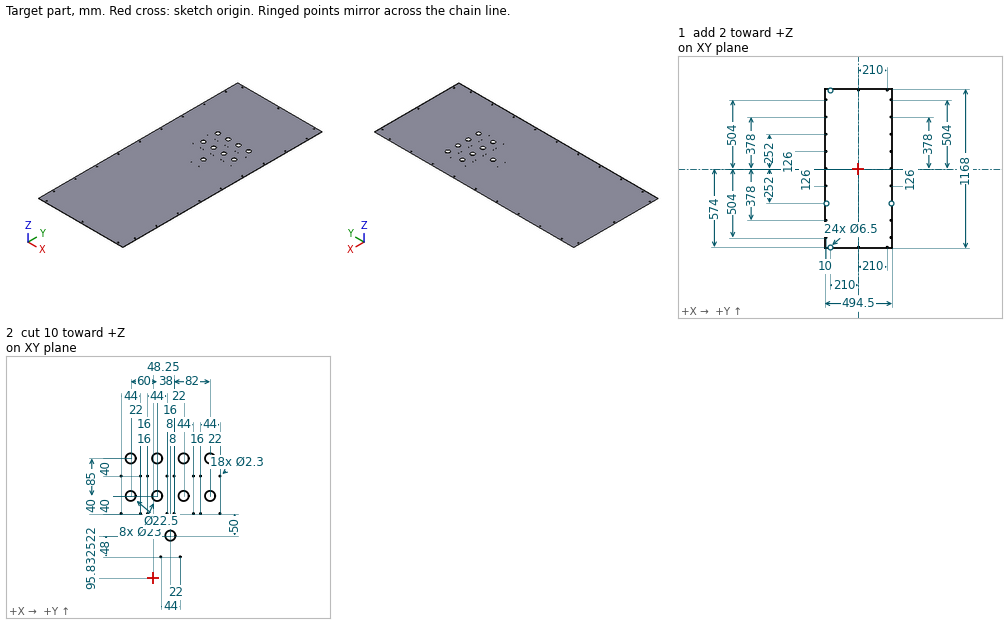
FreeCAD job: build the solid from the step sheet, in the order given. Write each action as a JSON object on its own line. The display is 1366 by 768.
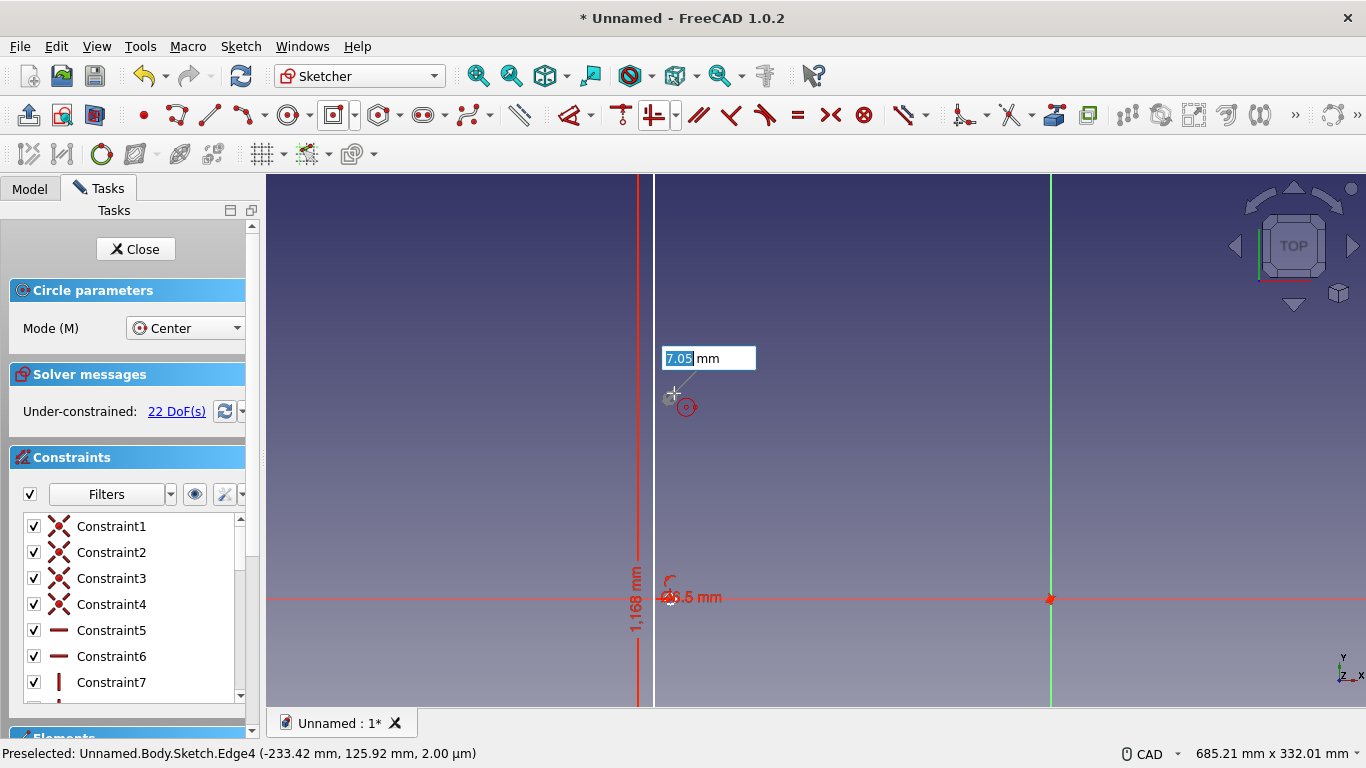
{"action": "type", "text": "6.5"}
{"action": "key", "text": "Return"}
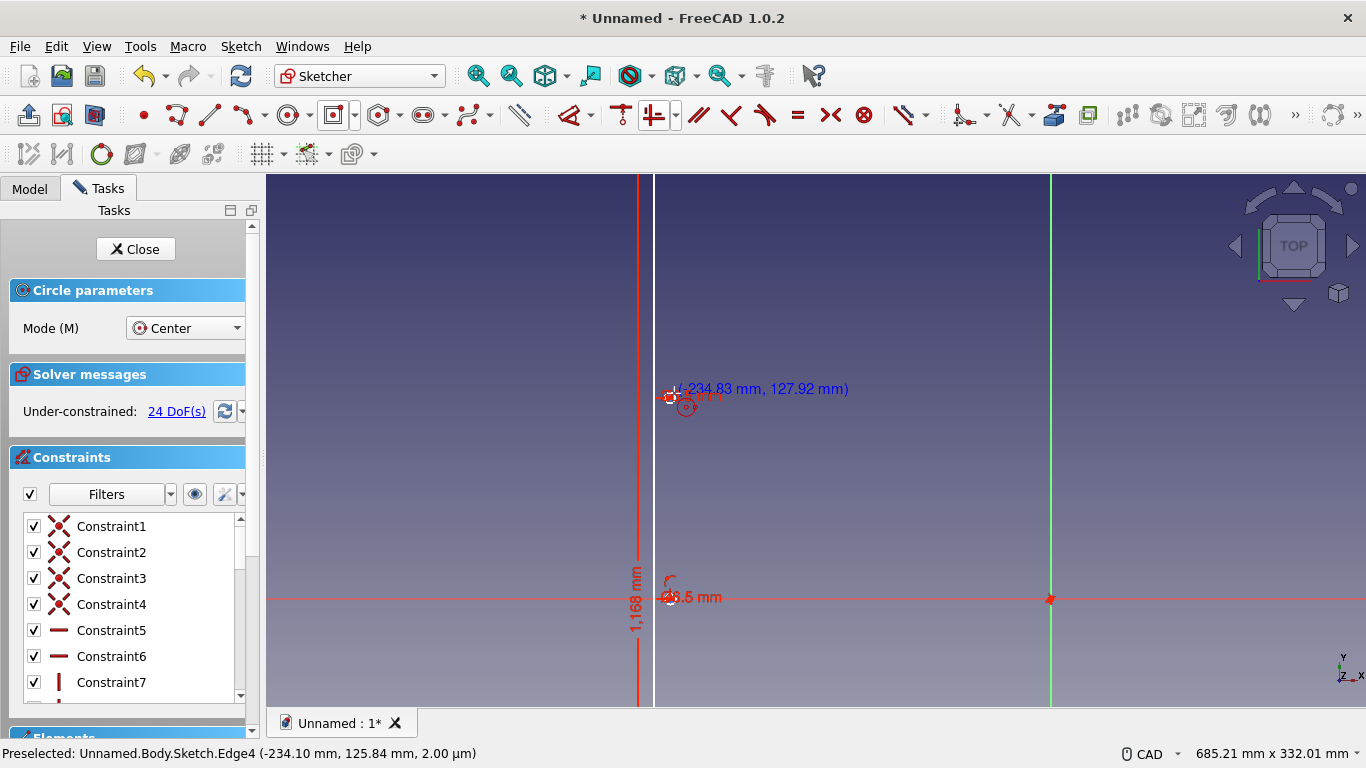
{"action": "scroll", "coordinate": [687, 409], "scroll_direction": "down", "scroll_amount": 9}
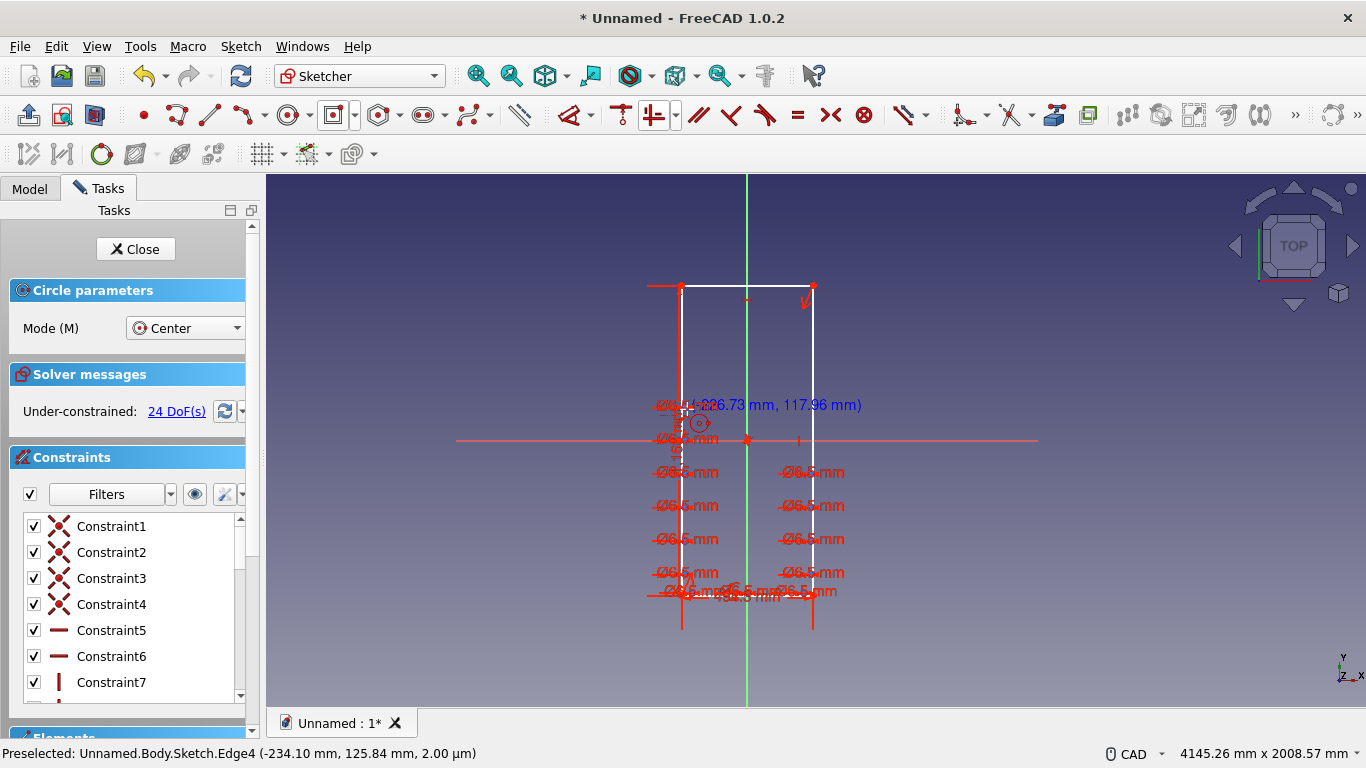
{"action": "scroll", "coordinate": [685, 374], "scroll_direction": "up", "scroll_amount": 17}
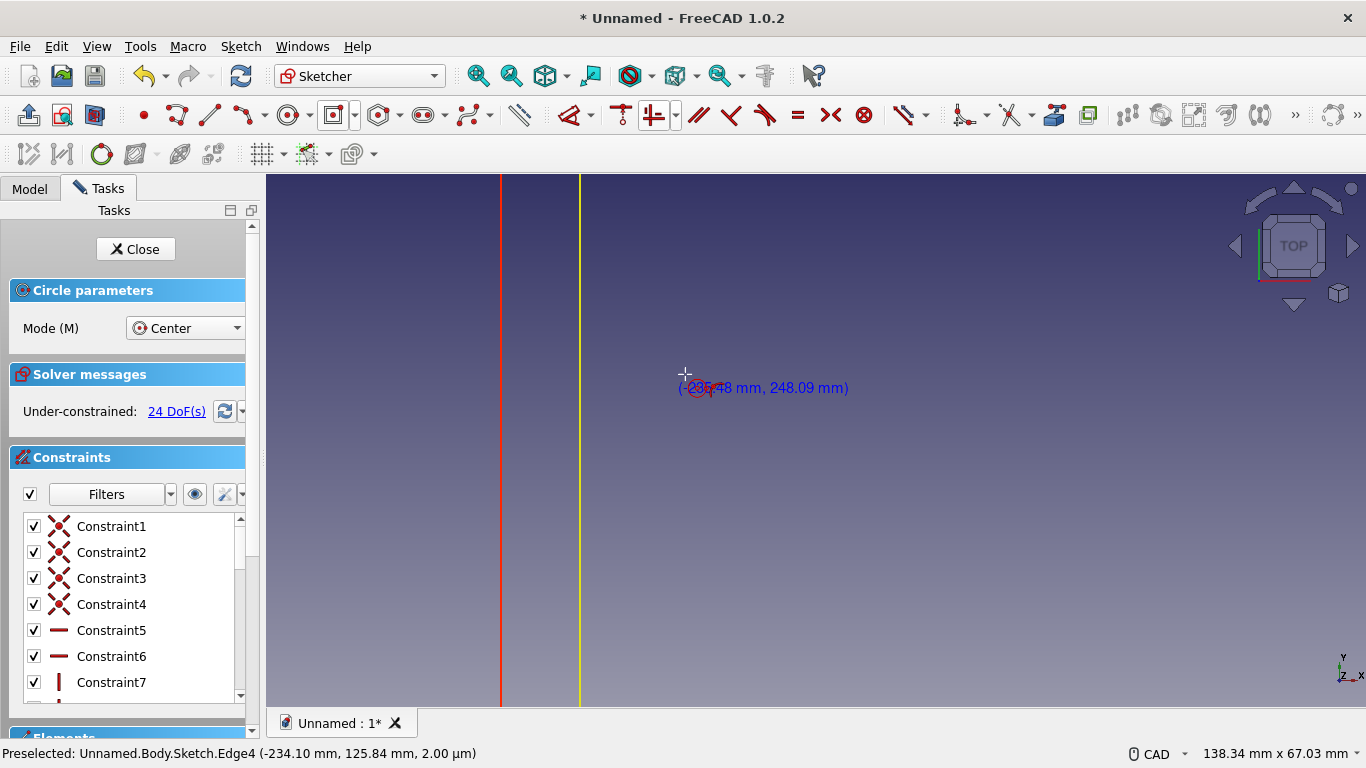
{"action": "scroll", "coordinate": [671, 359], "scroll_direction": "down", "scroll_amount": 16}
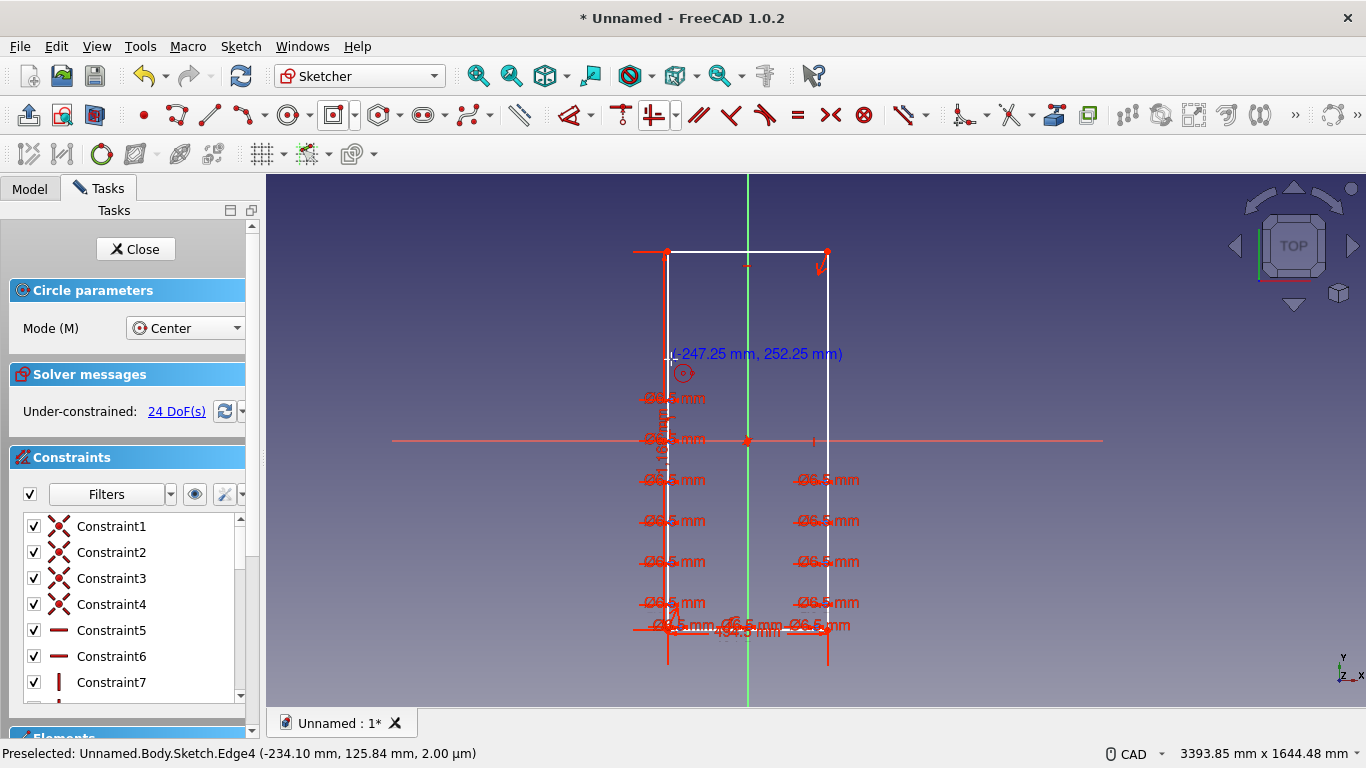
{"action": "scroll", "coordinate": [671, 359], "scroll_direction": "up", "scroll_amount": 8}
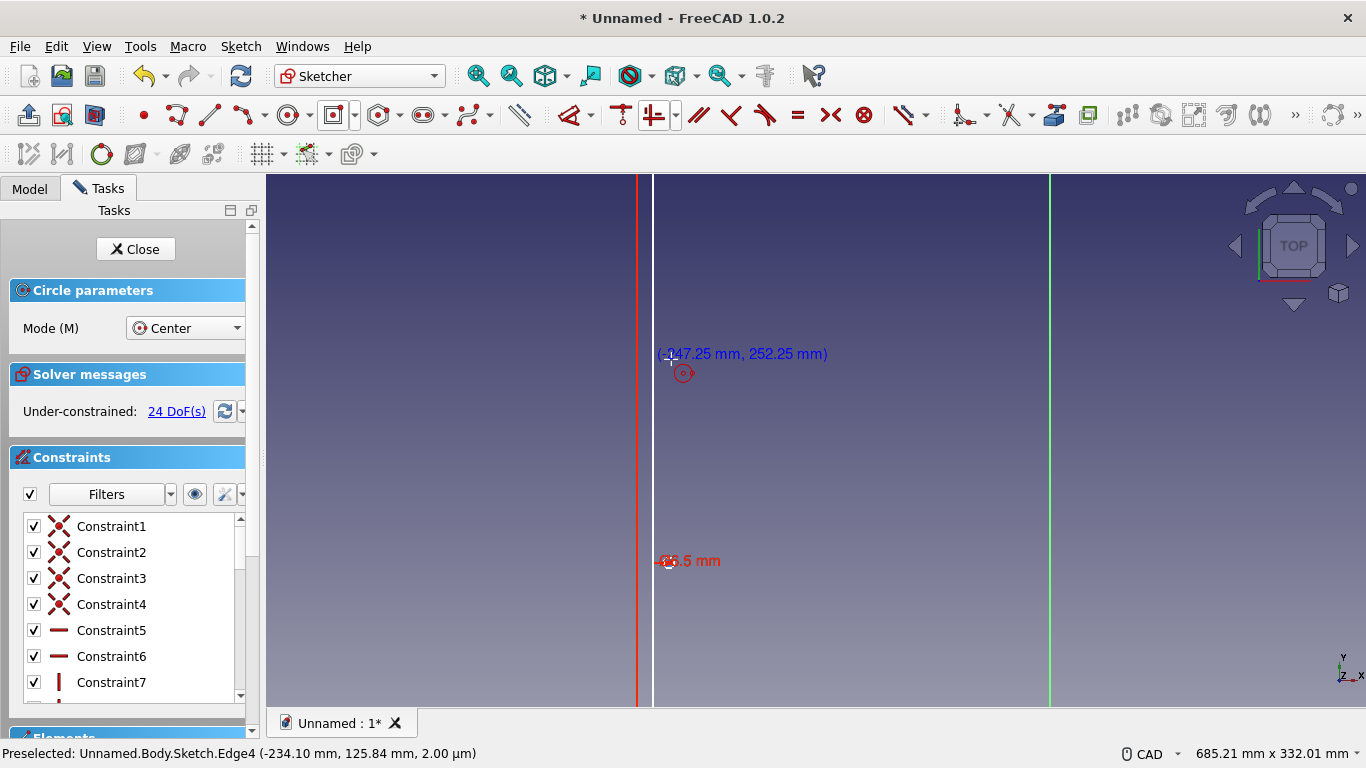
{"action": "left_click", "coordinate": [669, 360]}
{"action": "mouse_move", "coordinate": [673, 356]}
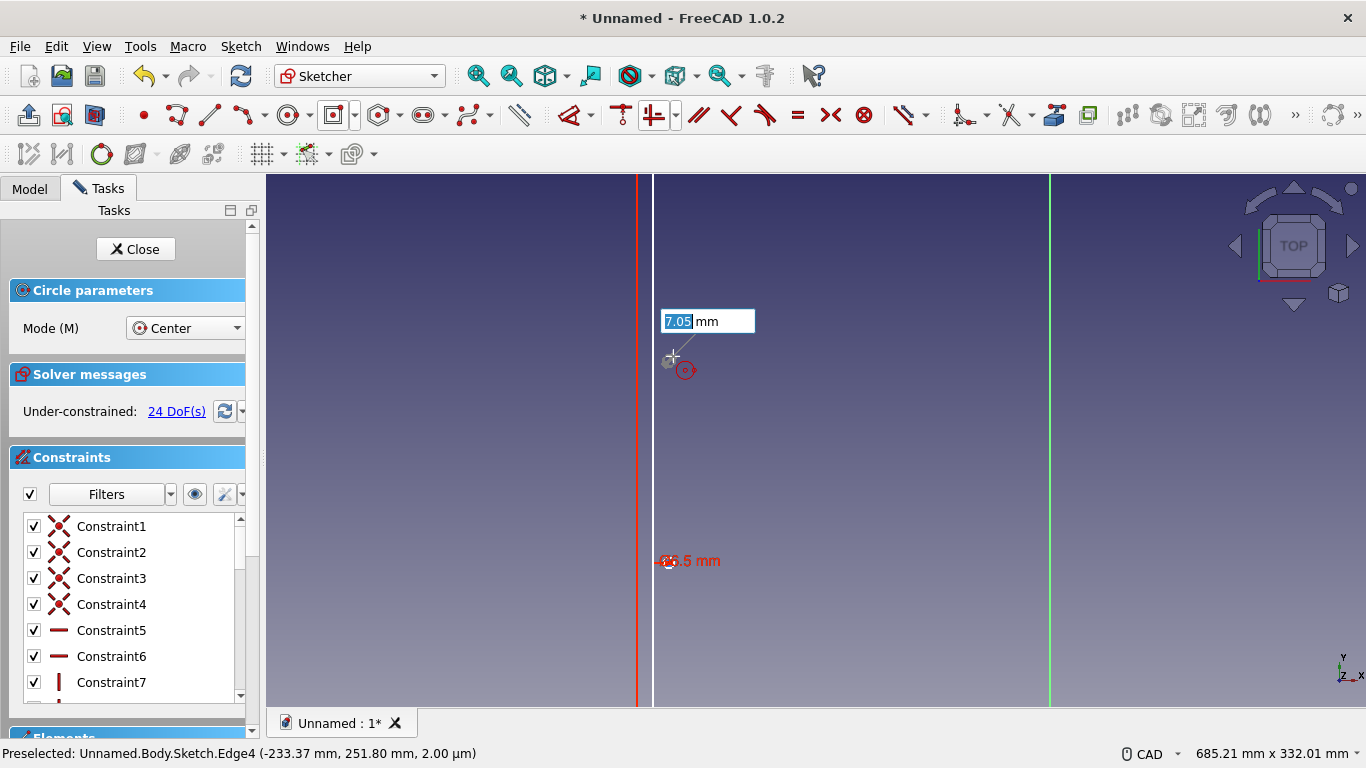
{"action": "type", "text": "6.5"}
{"action": "key", "text": "Return"}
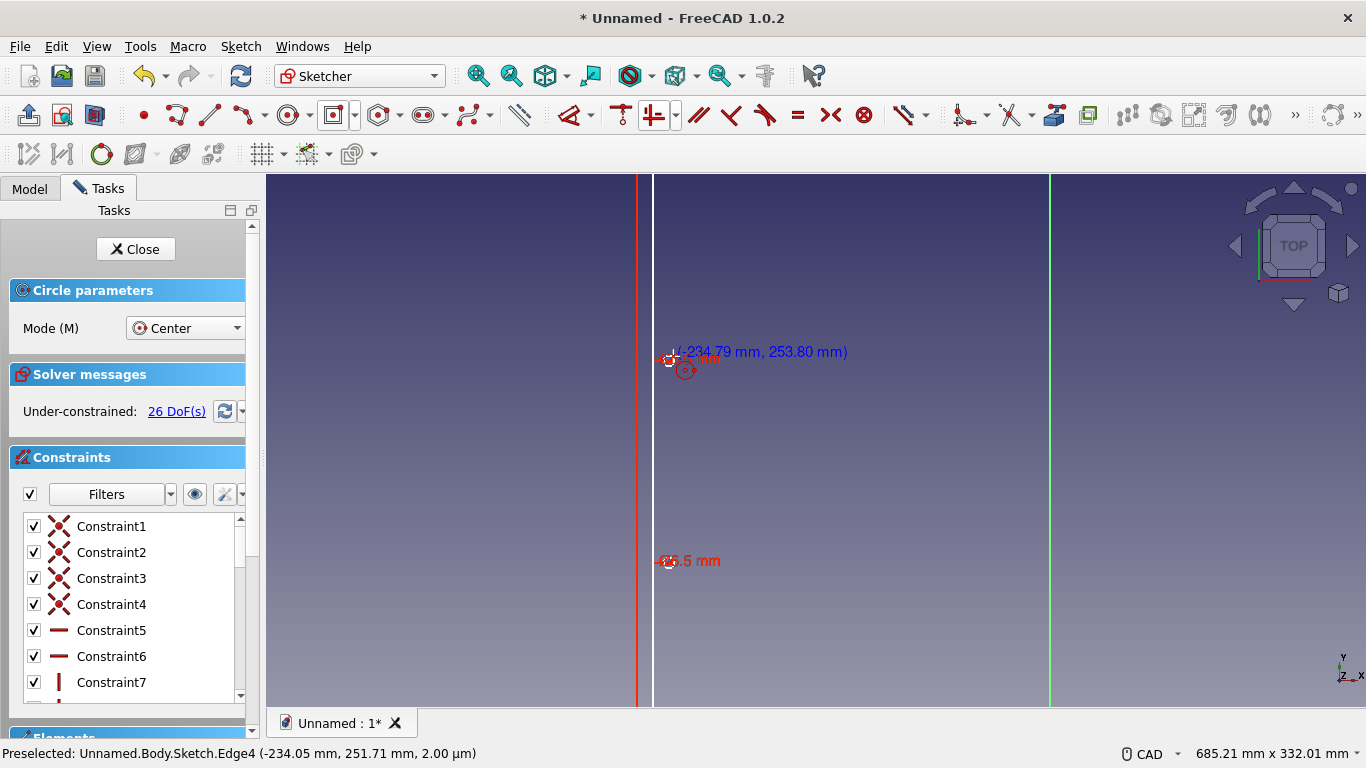
{"action": "scroll", "coordinate": [688, 376], "scroll_direction": "down", "scroll_amount": 9}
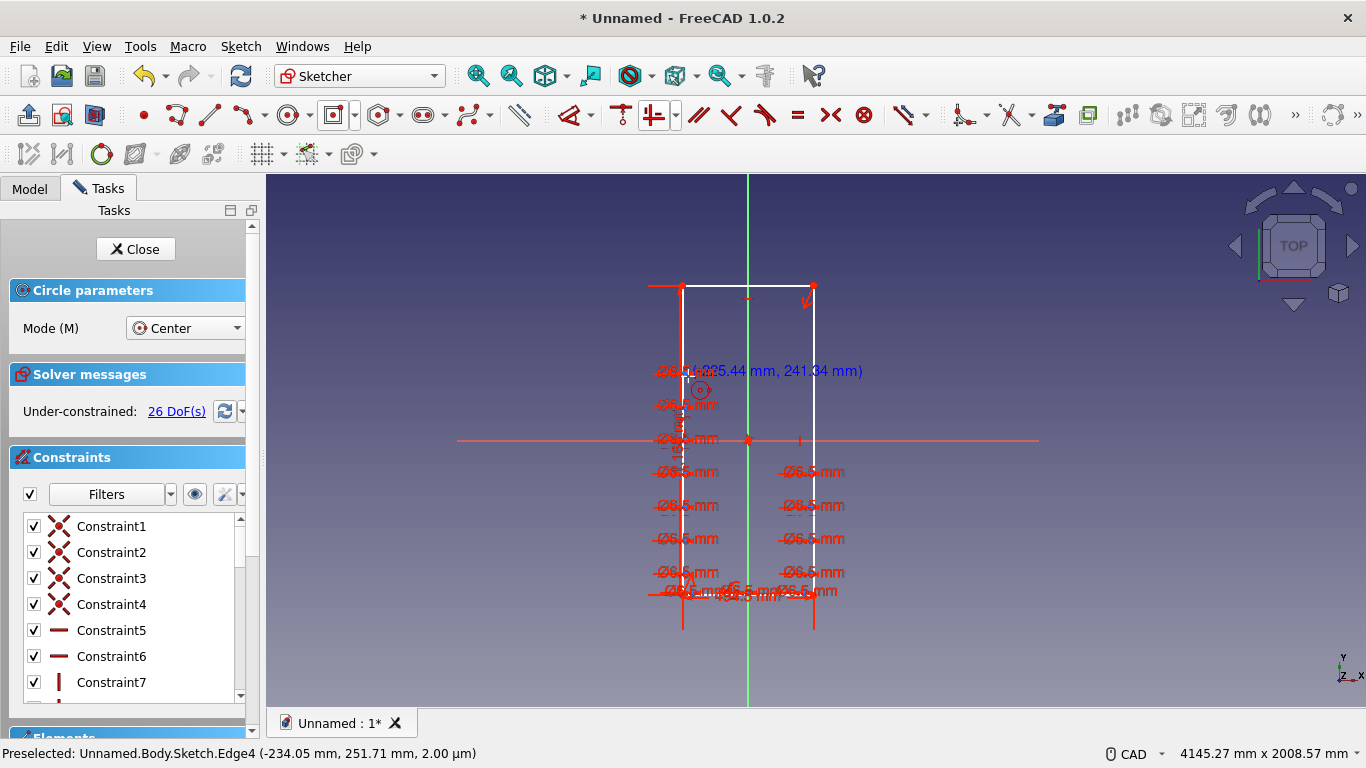
{"action": "scroll", "coordinate": [685, 340], "scroll_direction": "up", "scroll_amount": 17}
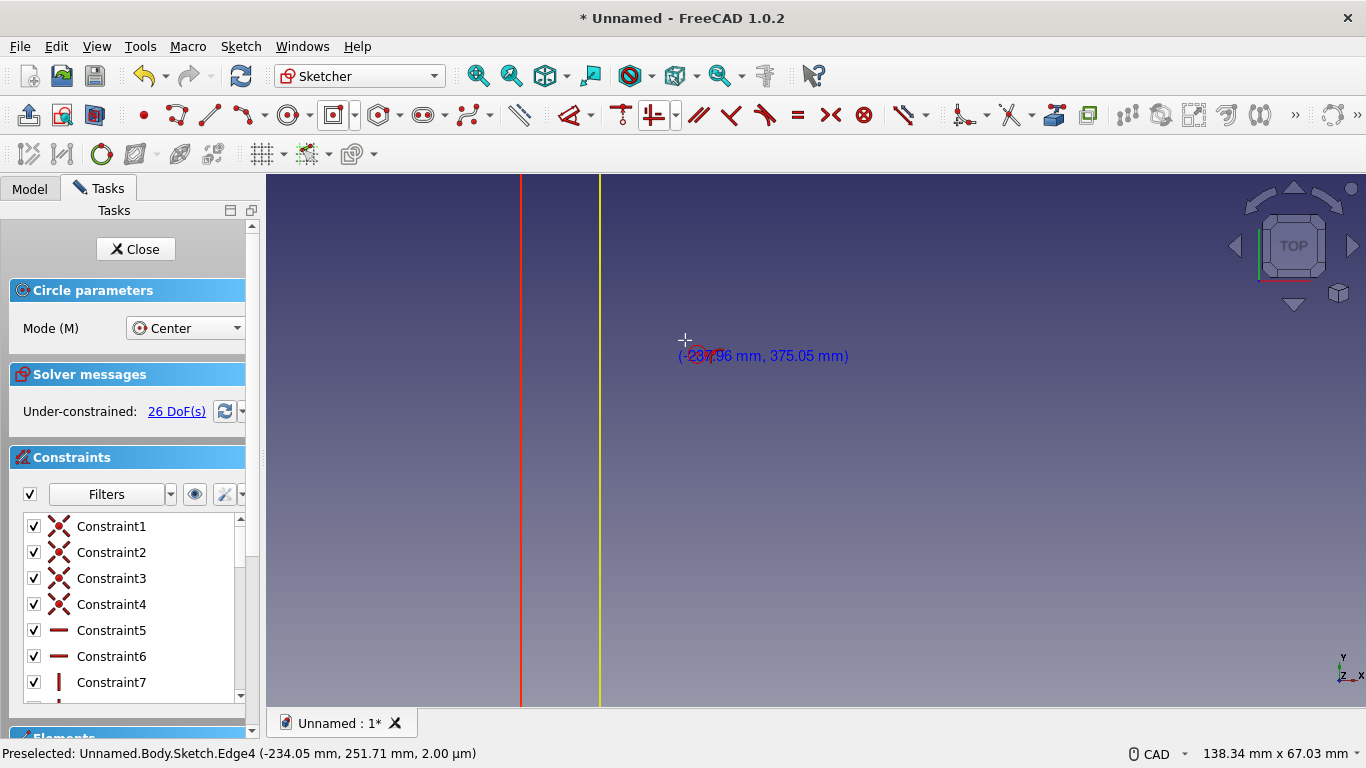
{"action": "scroll", "coordinate": [670, 317], "scroll_direction": "down", "scroll_amount": 16}